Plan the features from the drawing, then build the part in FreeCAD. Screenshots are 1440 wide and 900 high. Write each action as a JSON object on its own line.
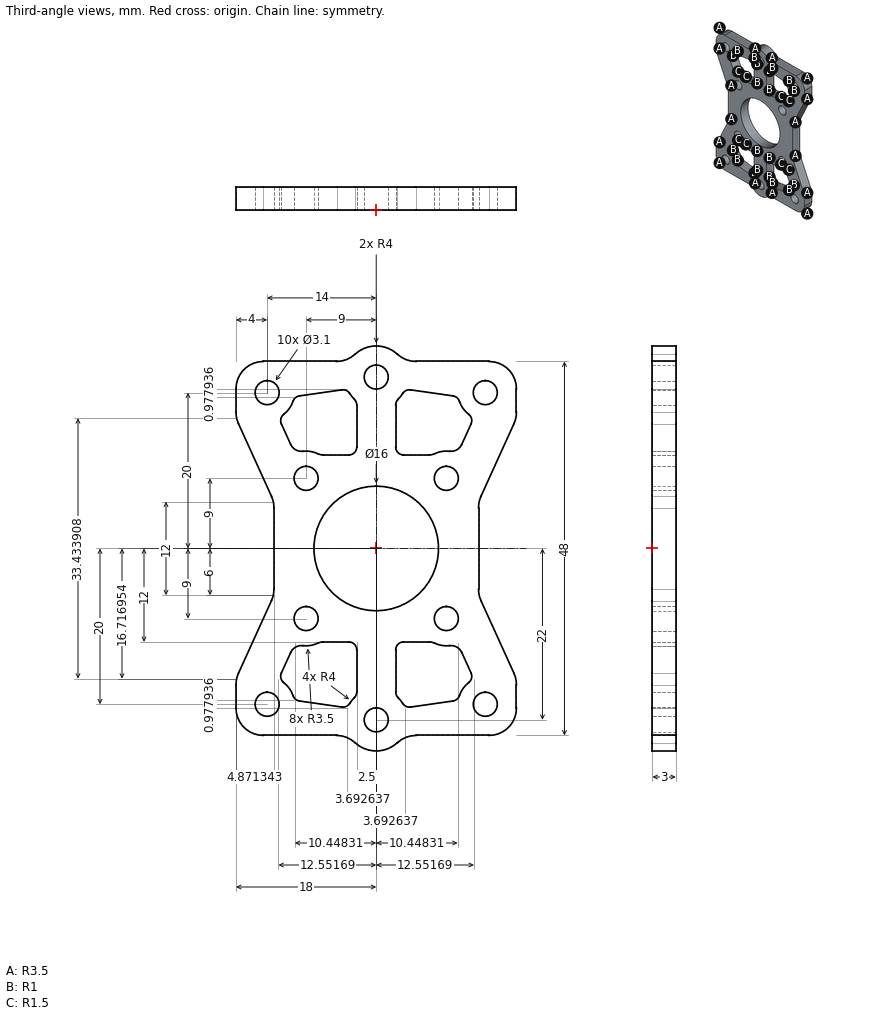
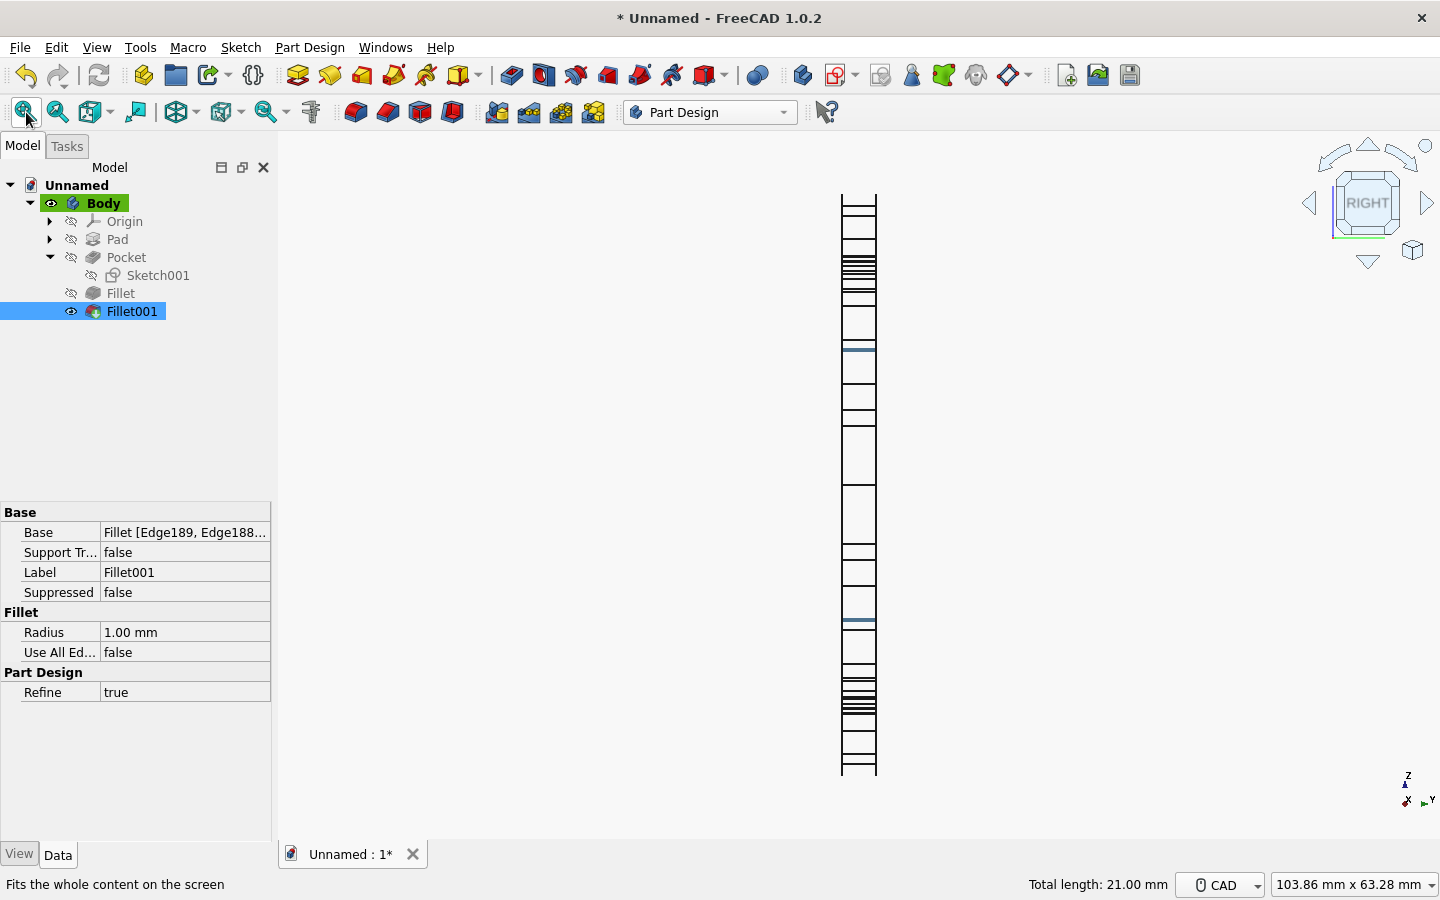
{"action": "key", "text": "5"}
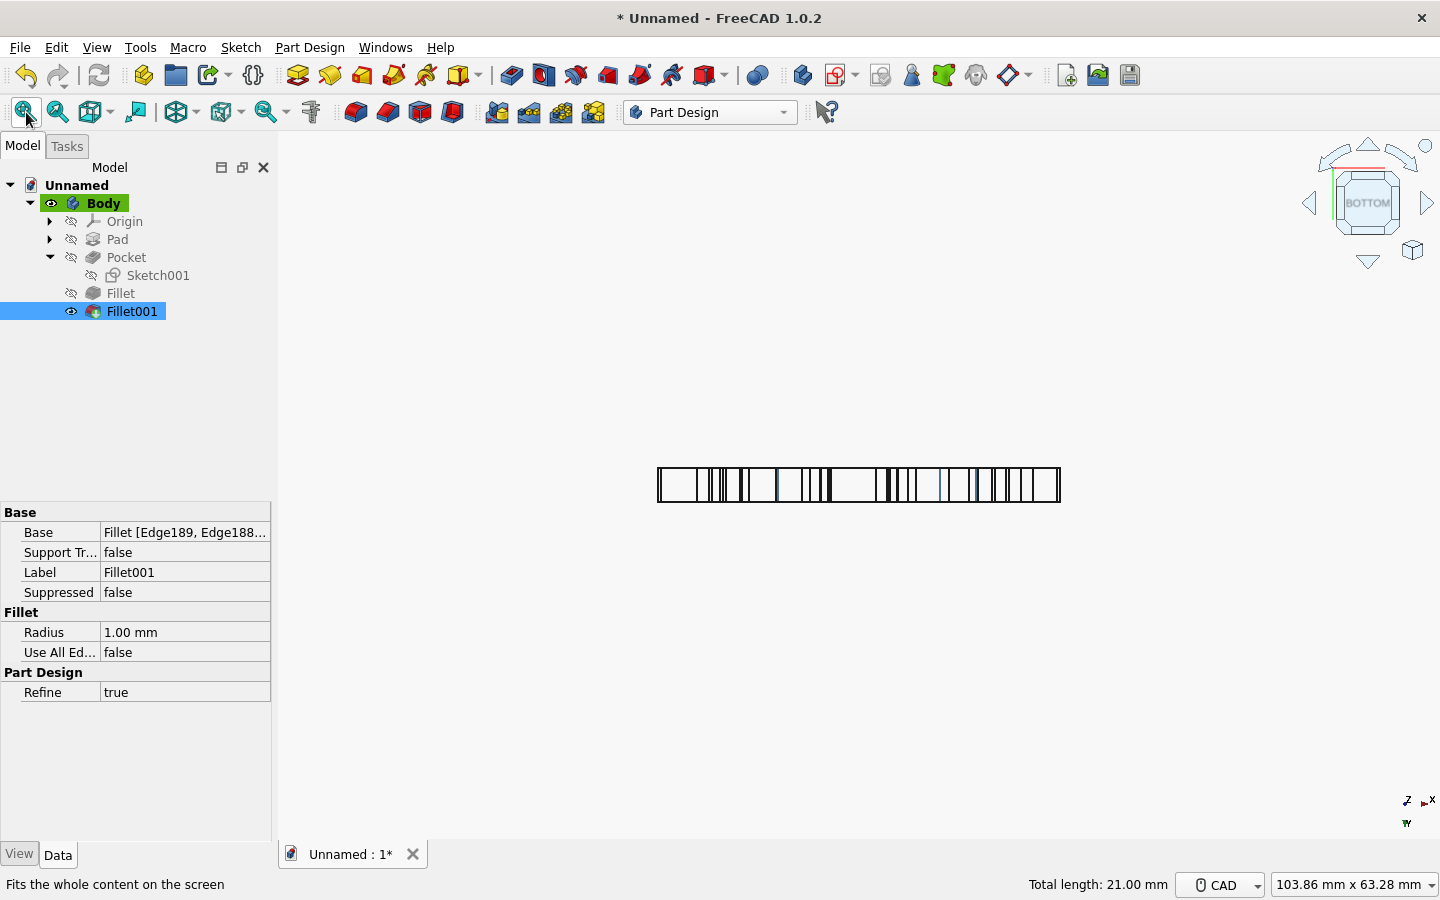
{"action": "key", "text": "v f"}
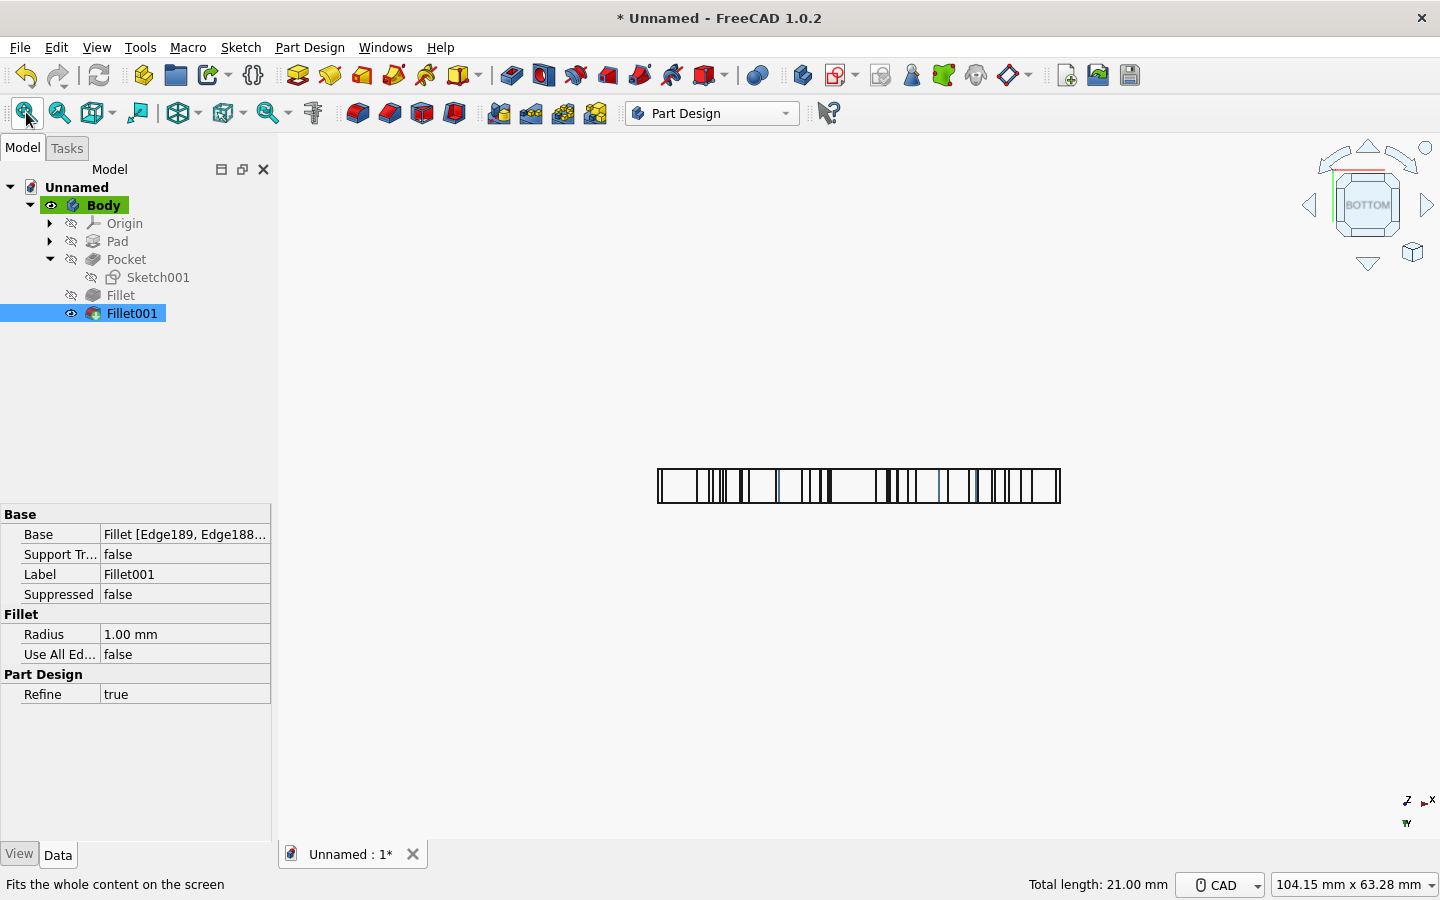
{"action": "key", "text": "4"}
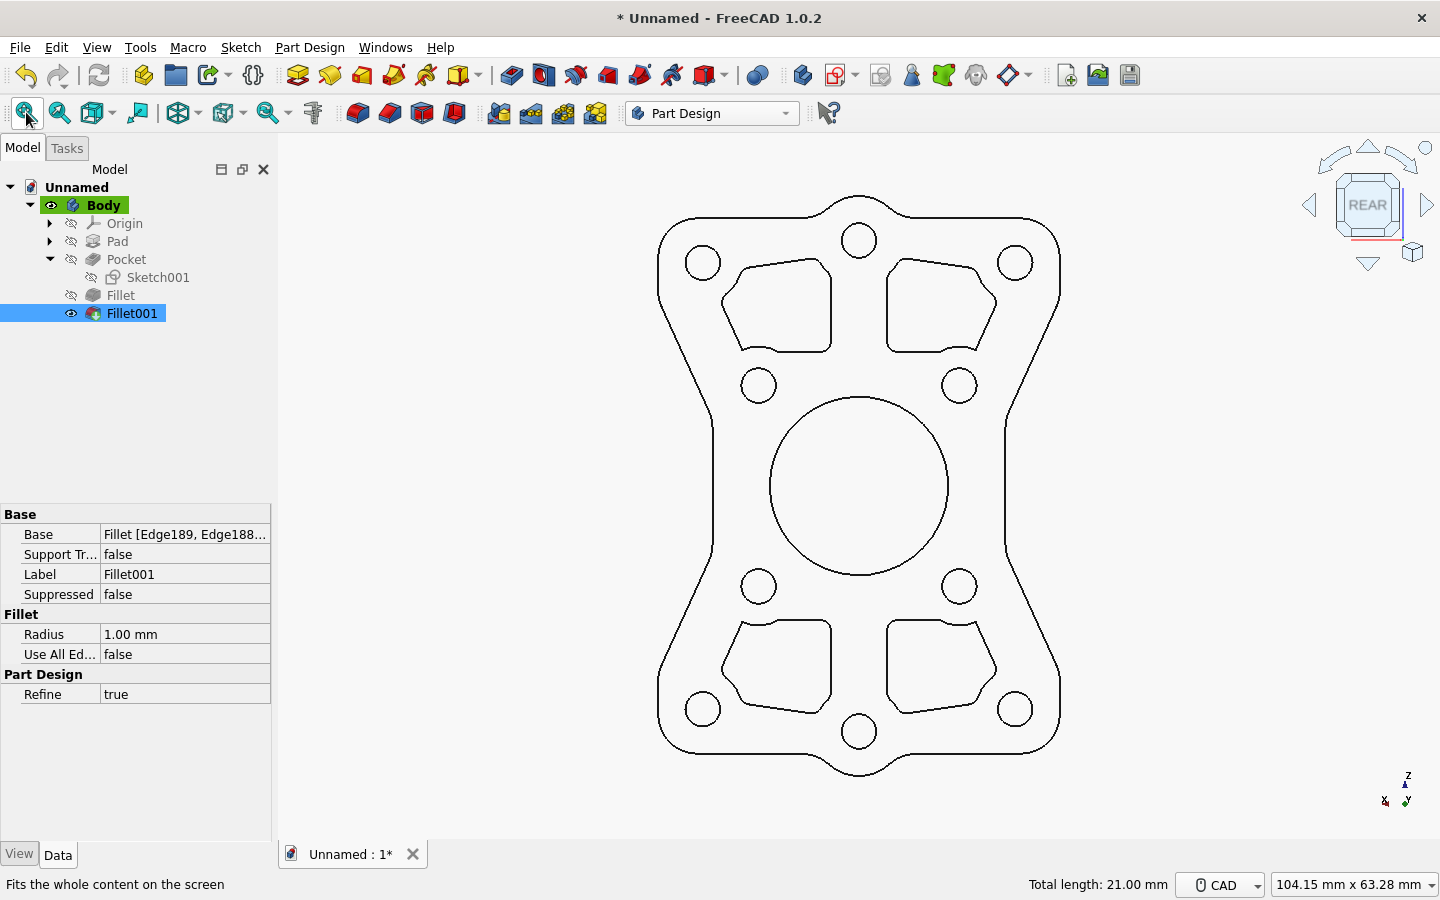
{"action": "key", "text": "6"}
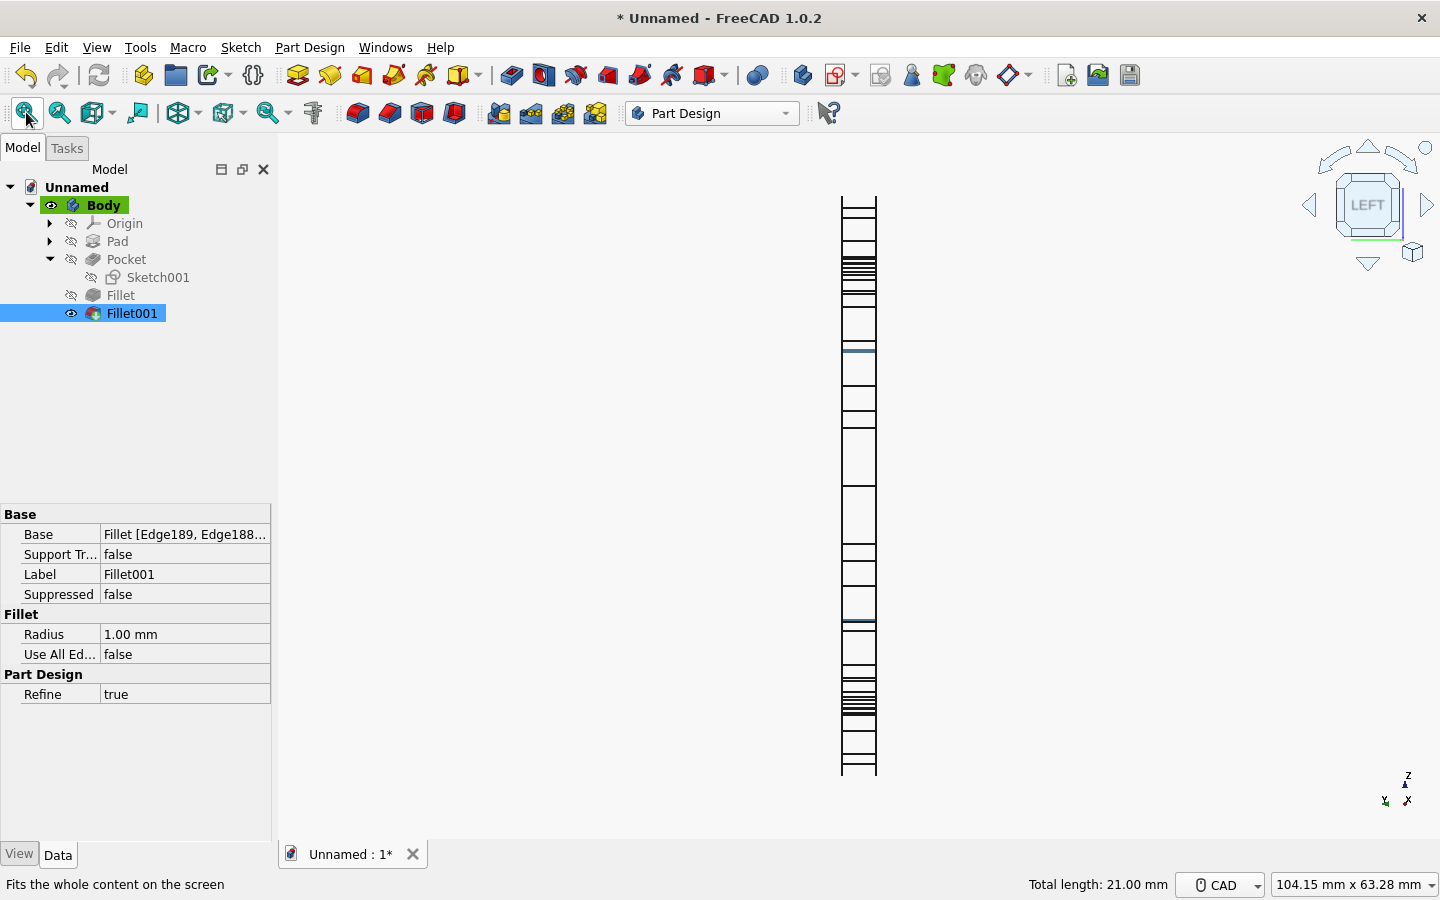
{"action": "left_click", "coordinate": [859, 621], "text": "ctrl"}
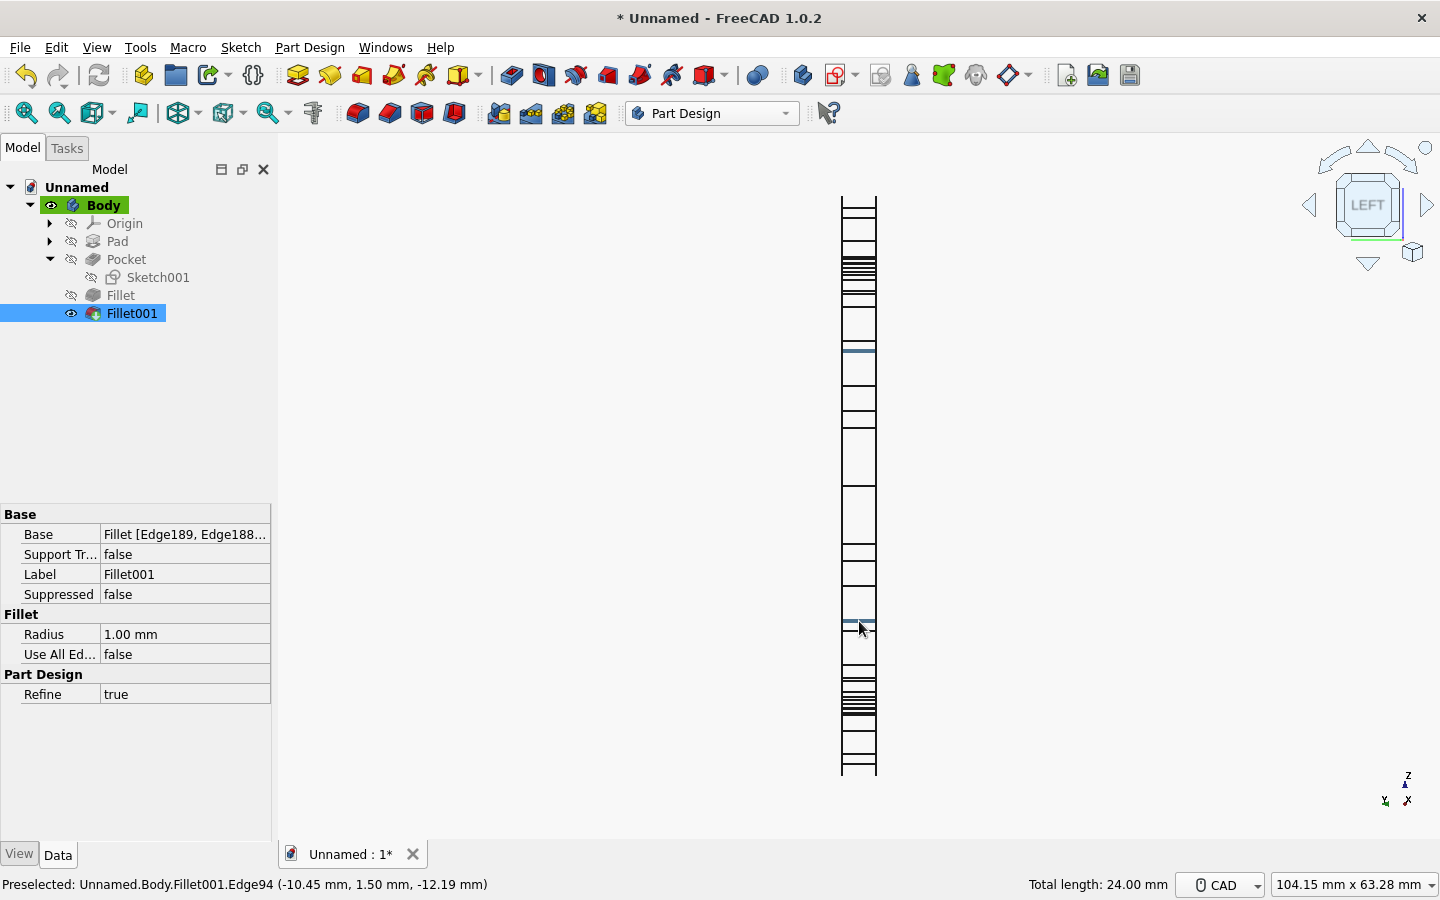
{"action": "key", "text": "v 1"}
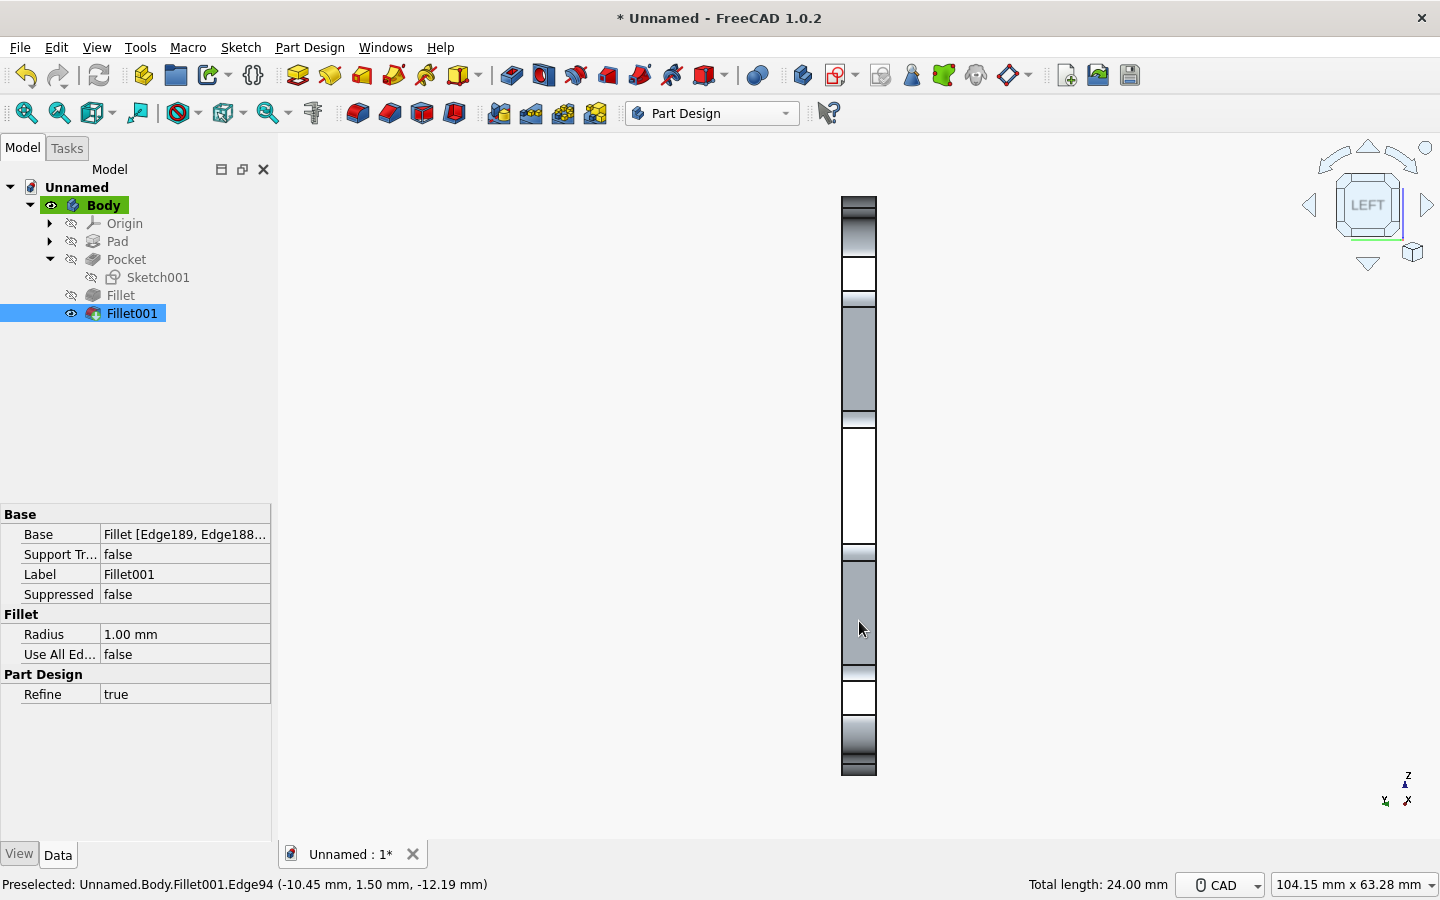
{"action": "left_click", "coordinate": [358, 114]}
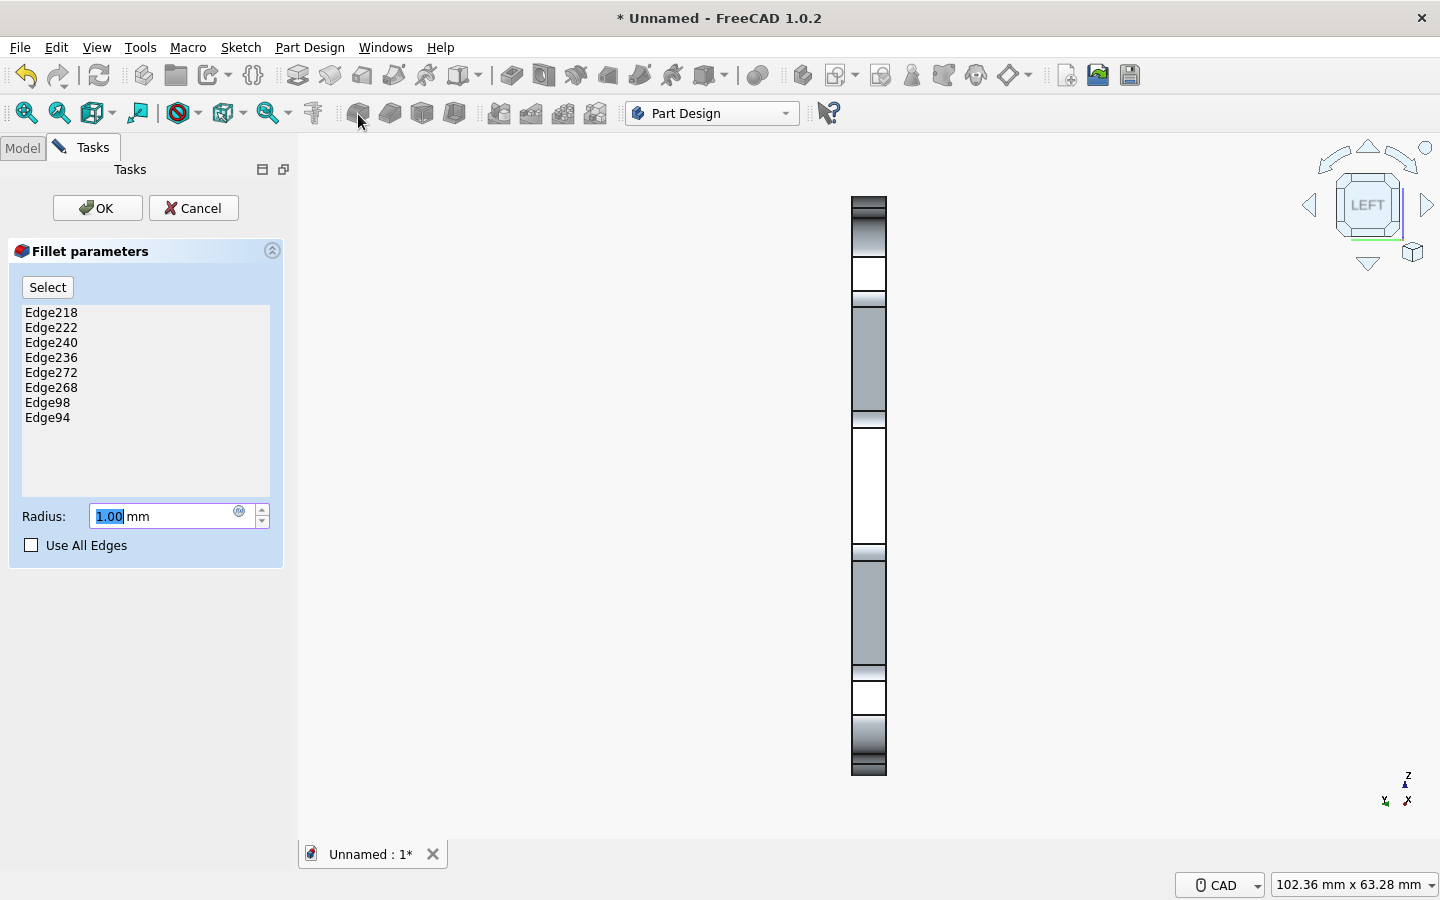
{"action": "type", "text": "1.5"}
{"action": "key", "text": "Tab"}